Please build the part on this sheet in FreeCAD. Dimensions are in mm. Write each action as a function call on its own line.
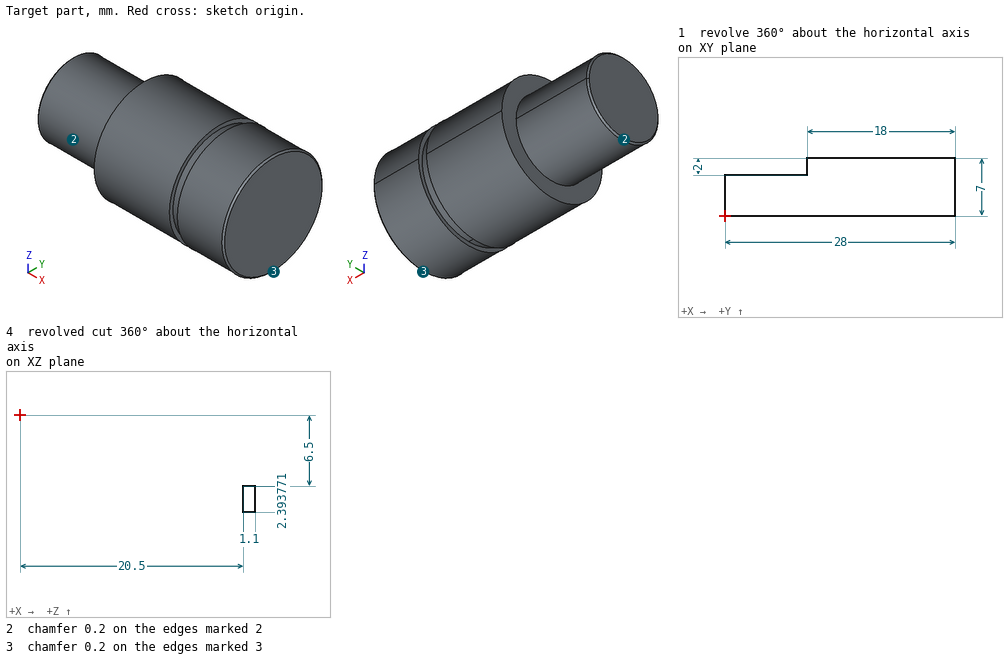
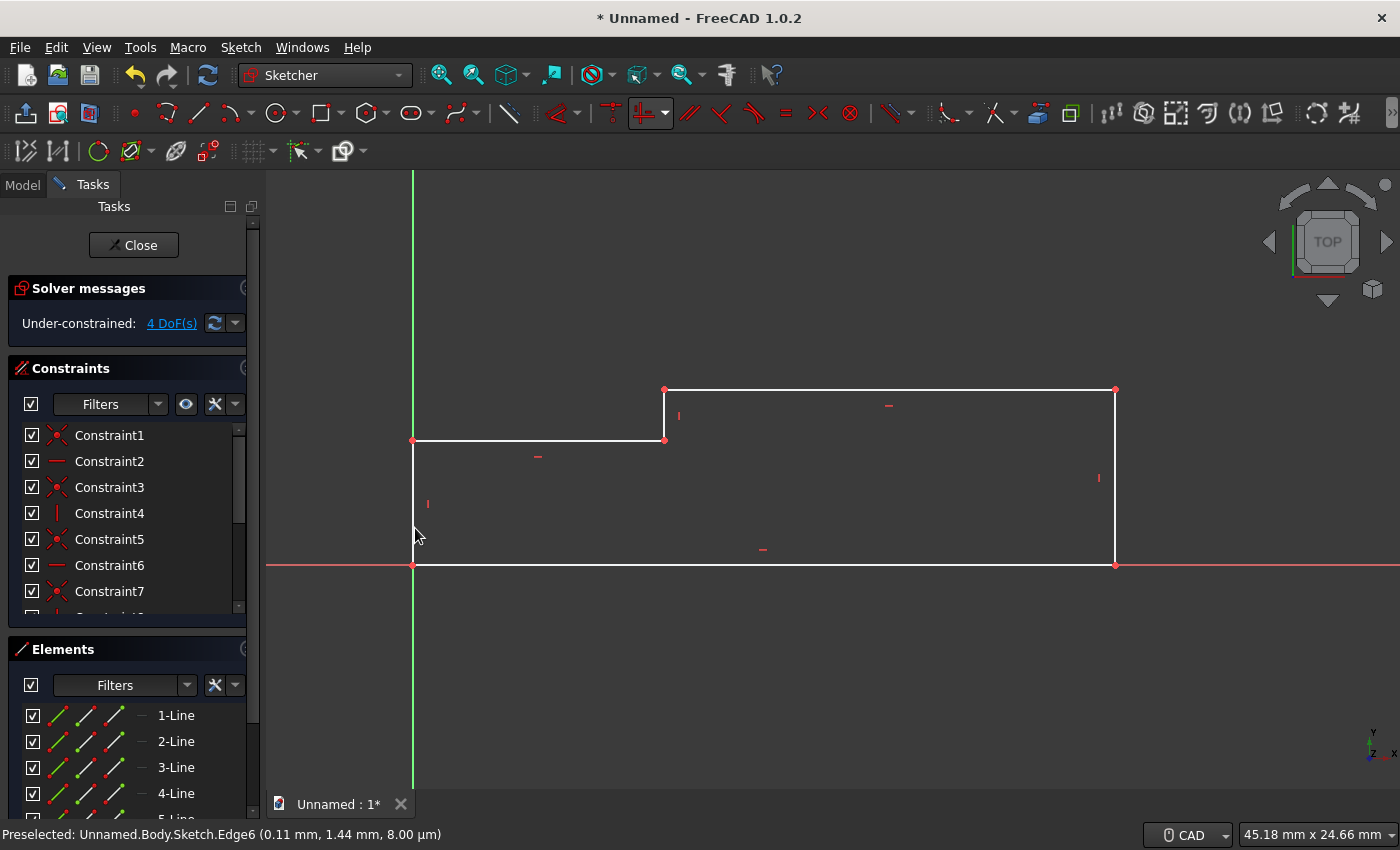
click(1115, 513)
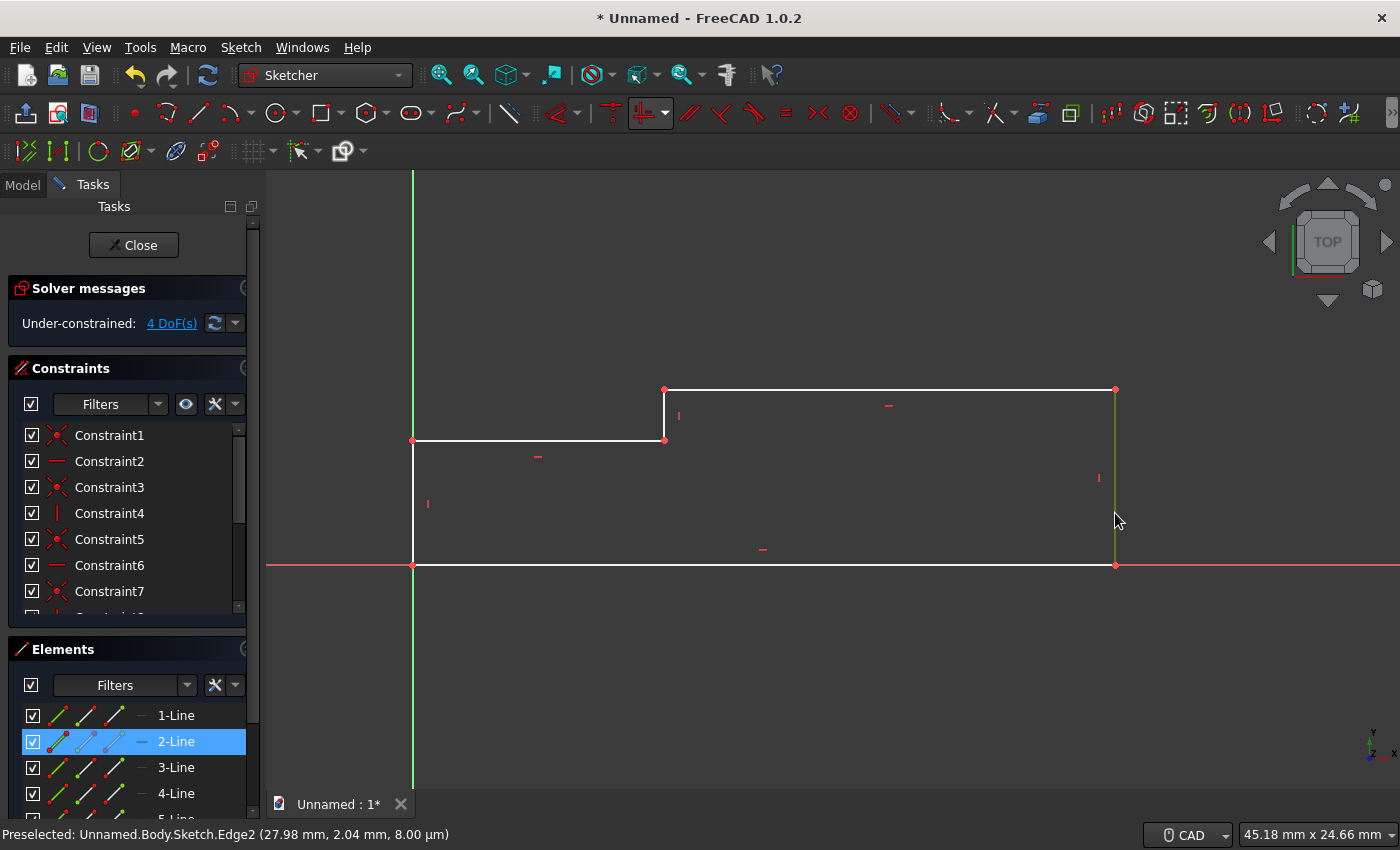
key(i)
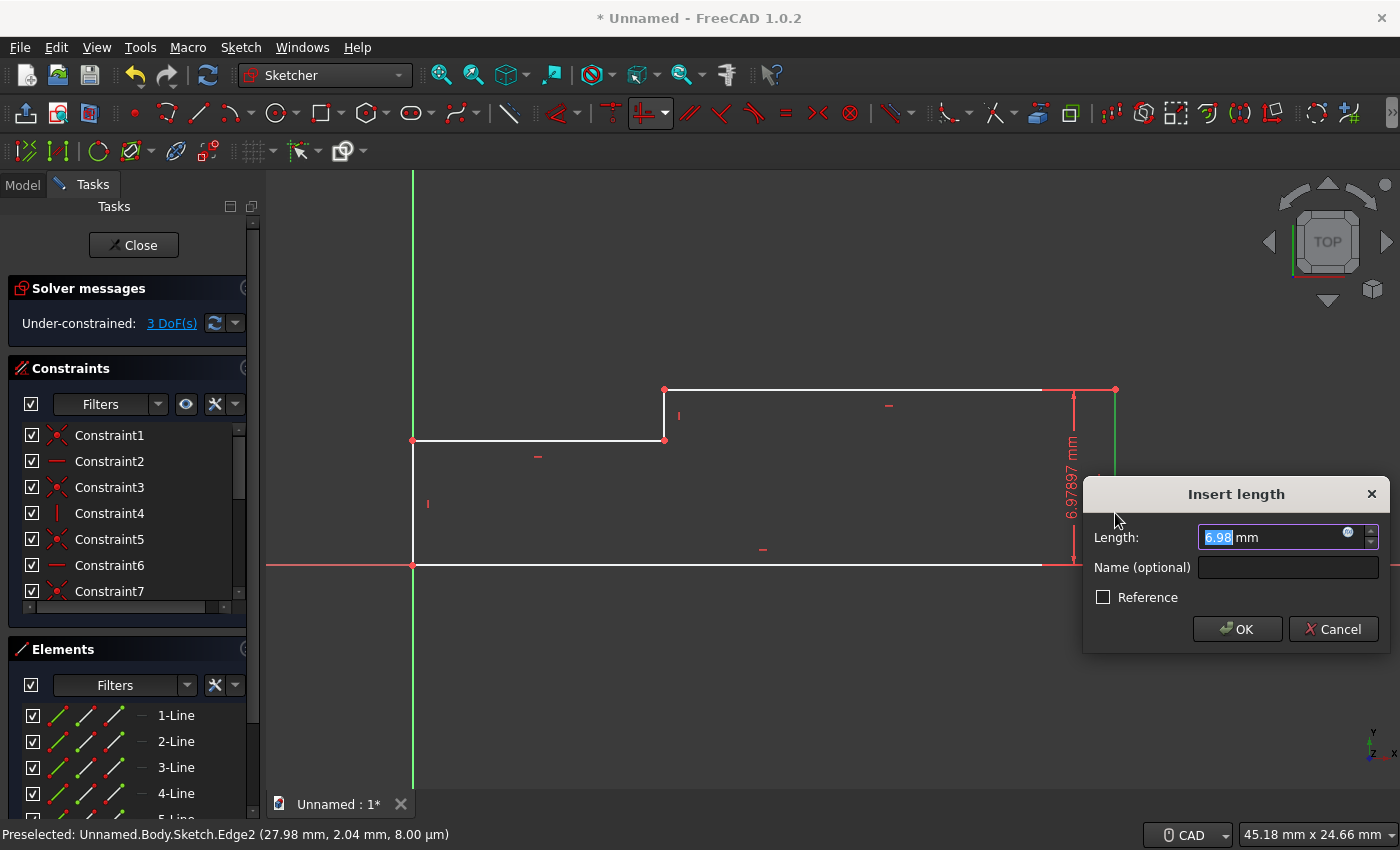
text(7)
key(Return)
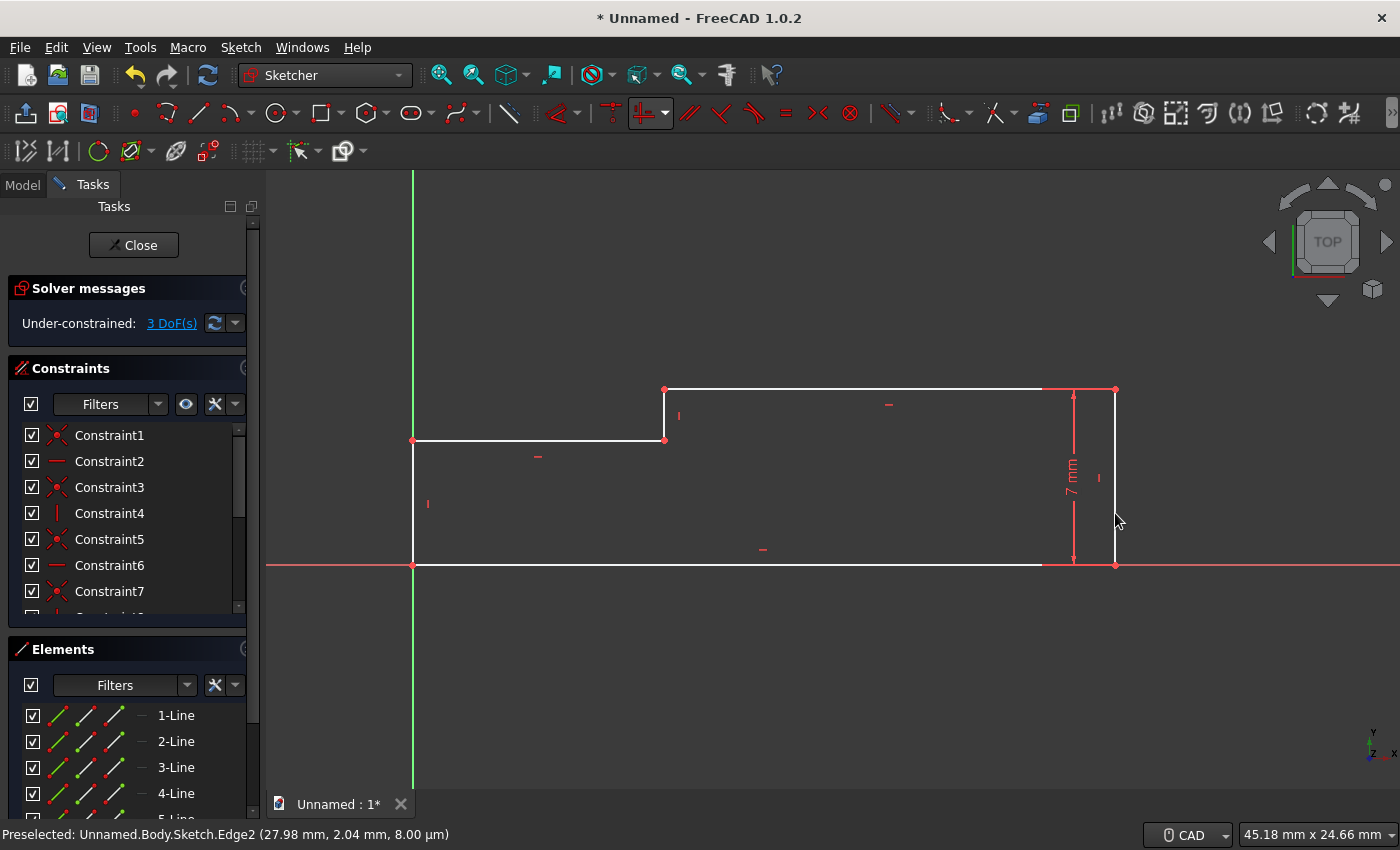
click(664, 405)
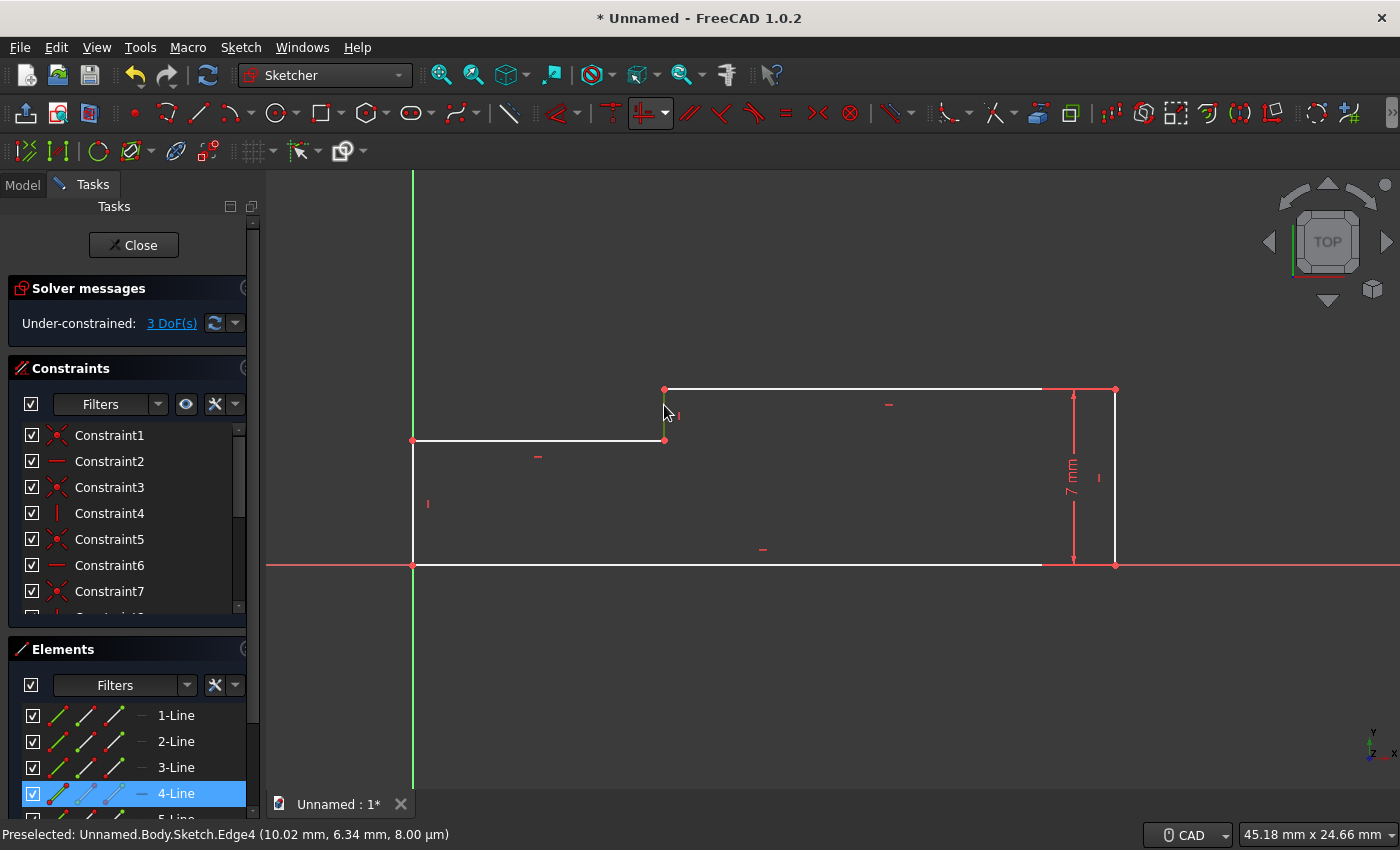
click(580, 114)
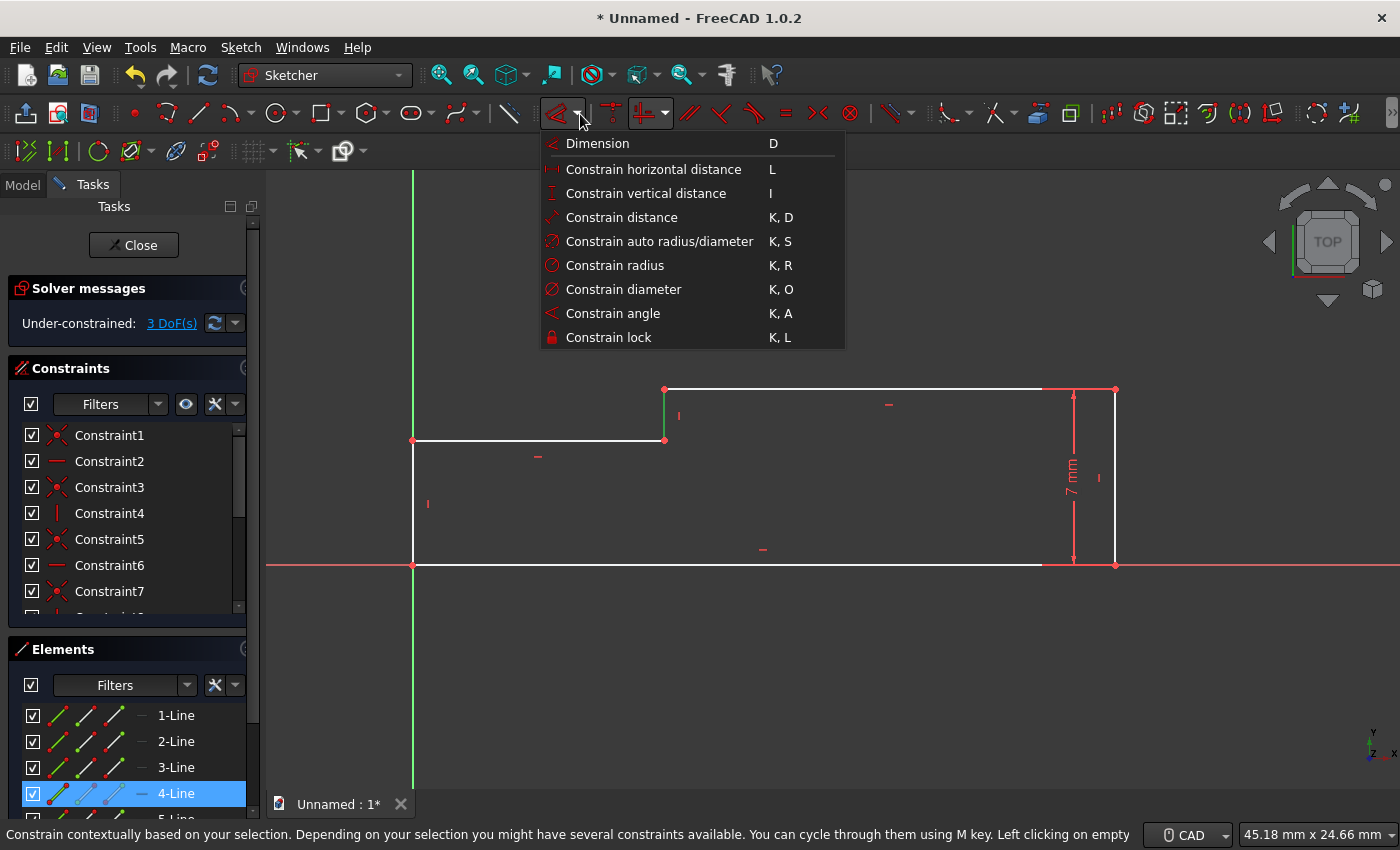
click(693, 193)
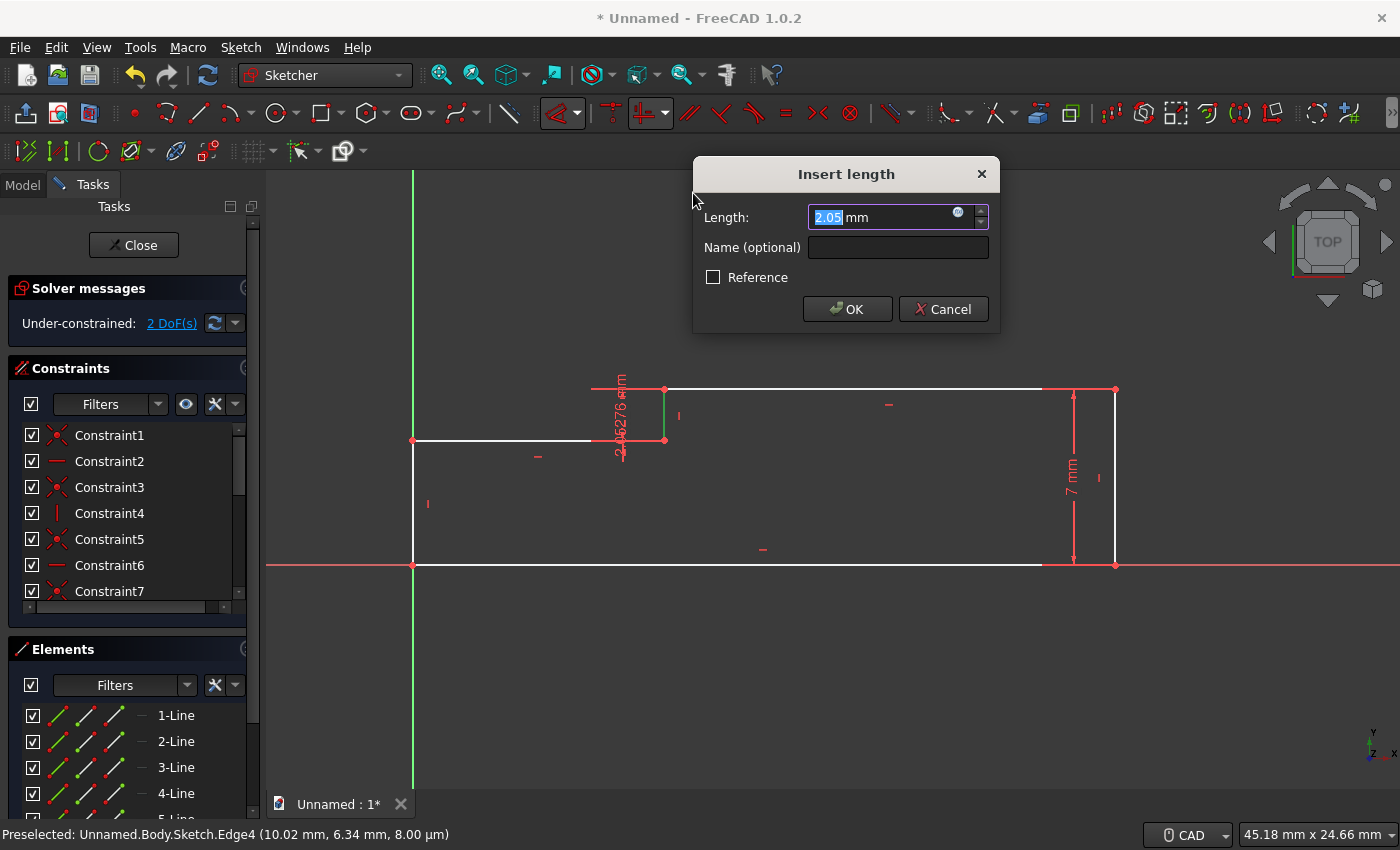
text(2)
key(Return)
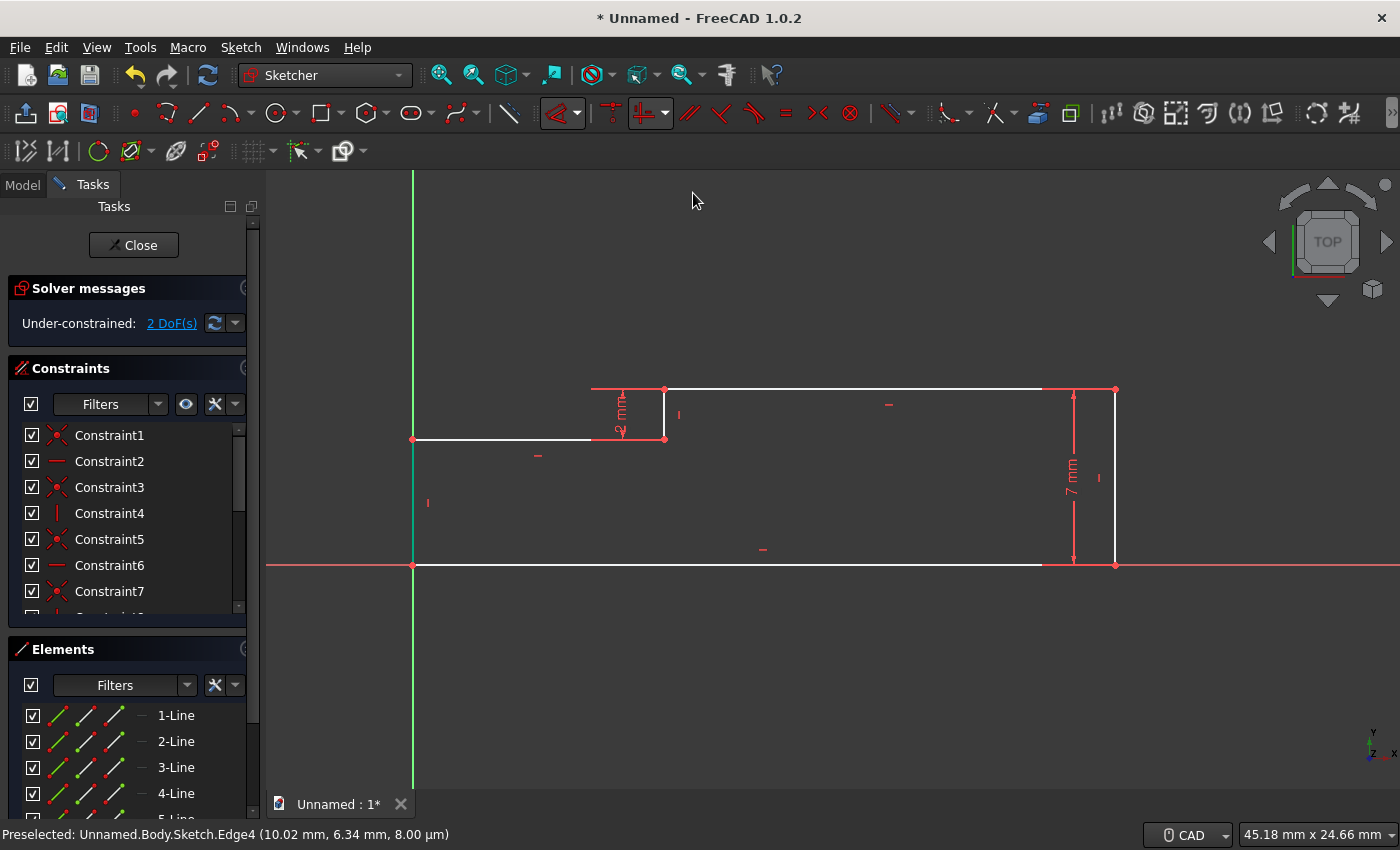
click(623, 565)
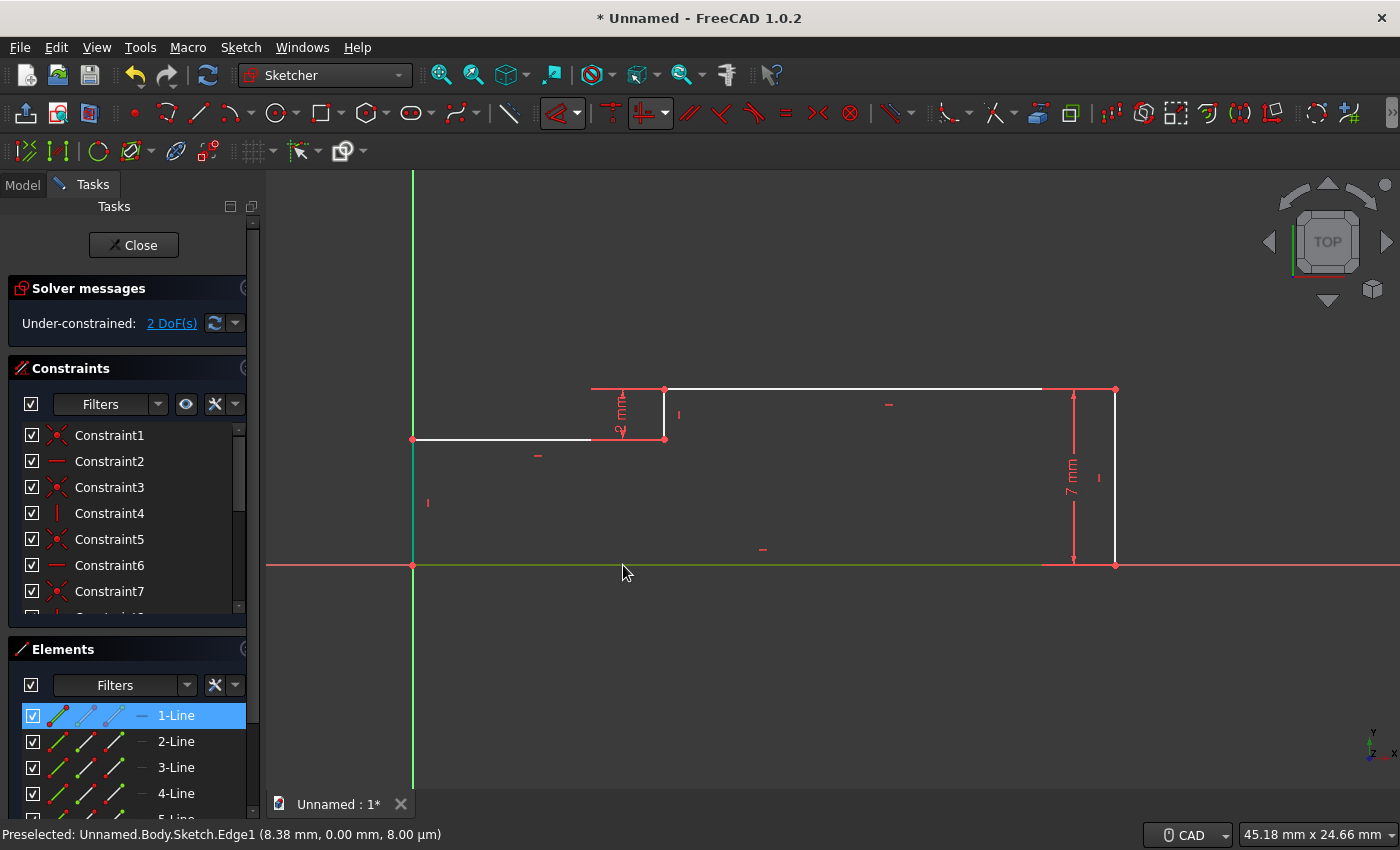
key(l)